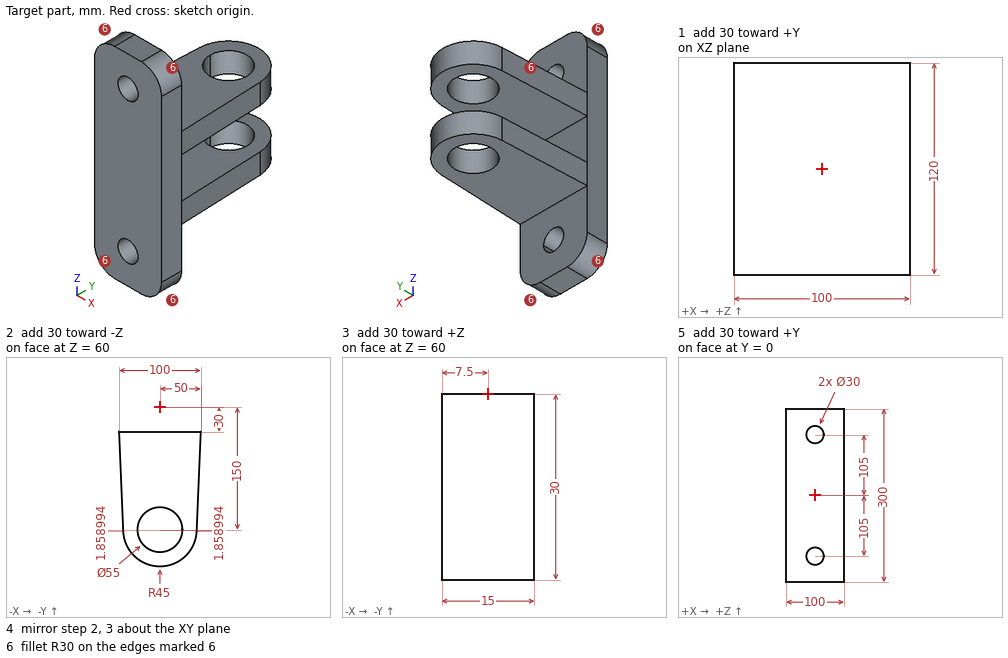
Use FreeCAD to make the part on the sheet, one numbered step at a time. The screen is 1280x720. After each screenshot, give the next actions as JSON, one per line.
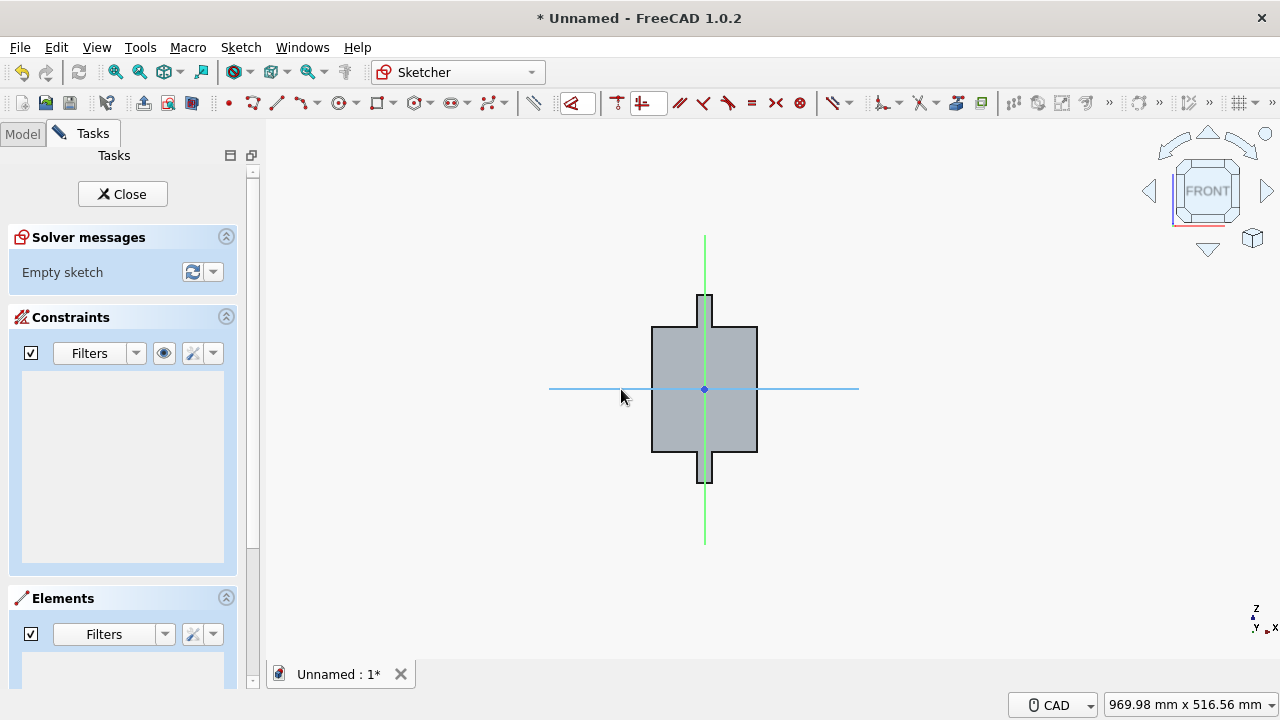
{"action": "left_click", "coordinate": [396, 104]}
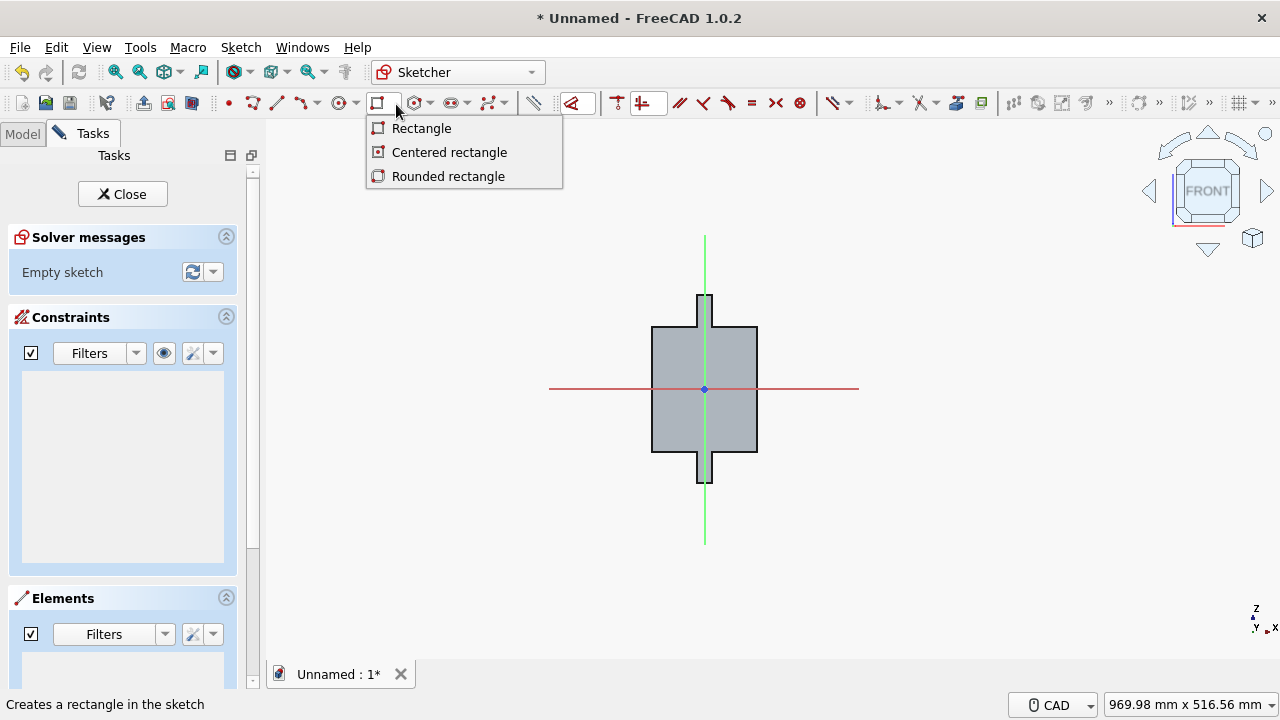
{"action": "left_click", "coordinate": [464, 152]}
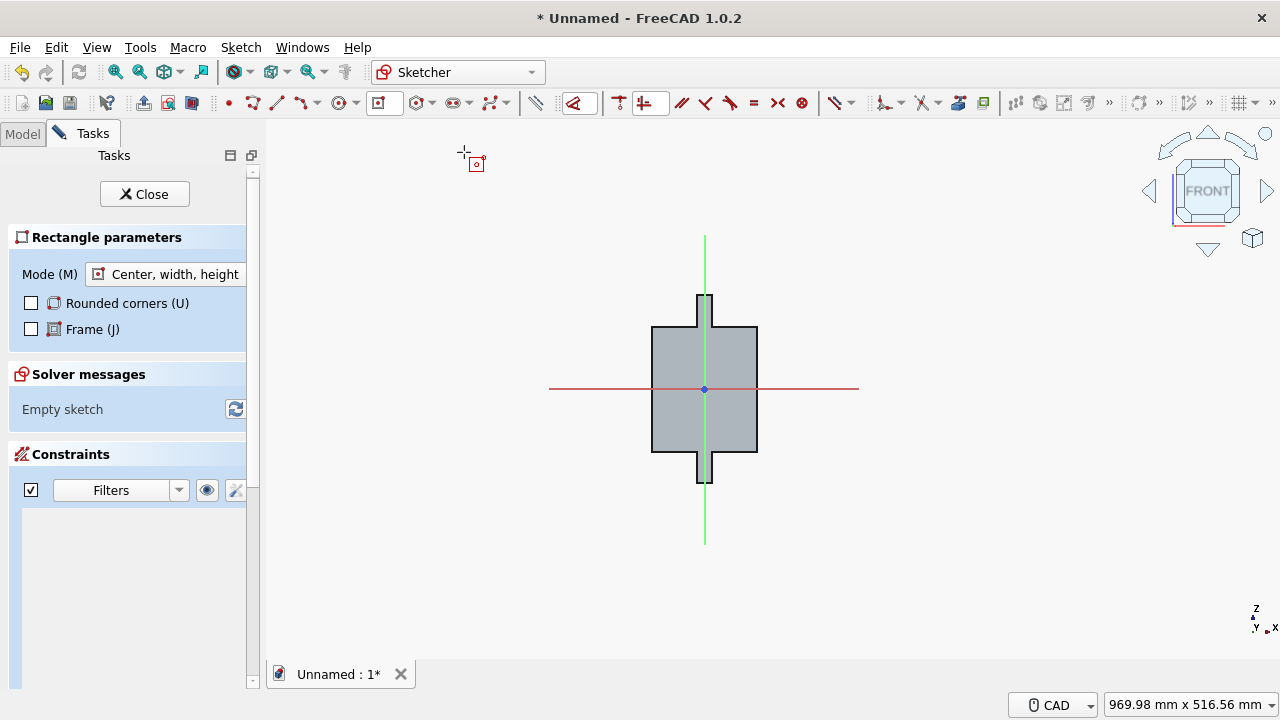
{"action": "left_click", "coordinate": [705, 389]}
{"action": "mouse_move", "coordinate": [757, 232]}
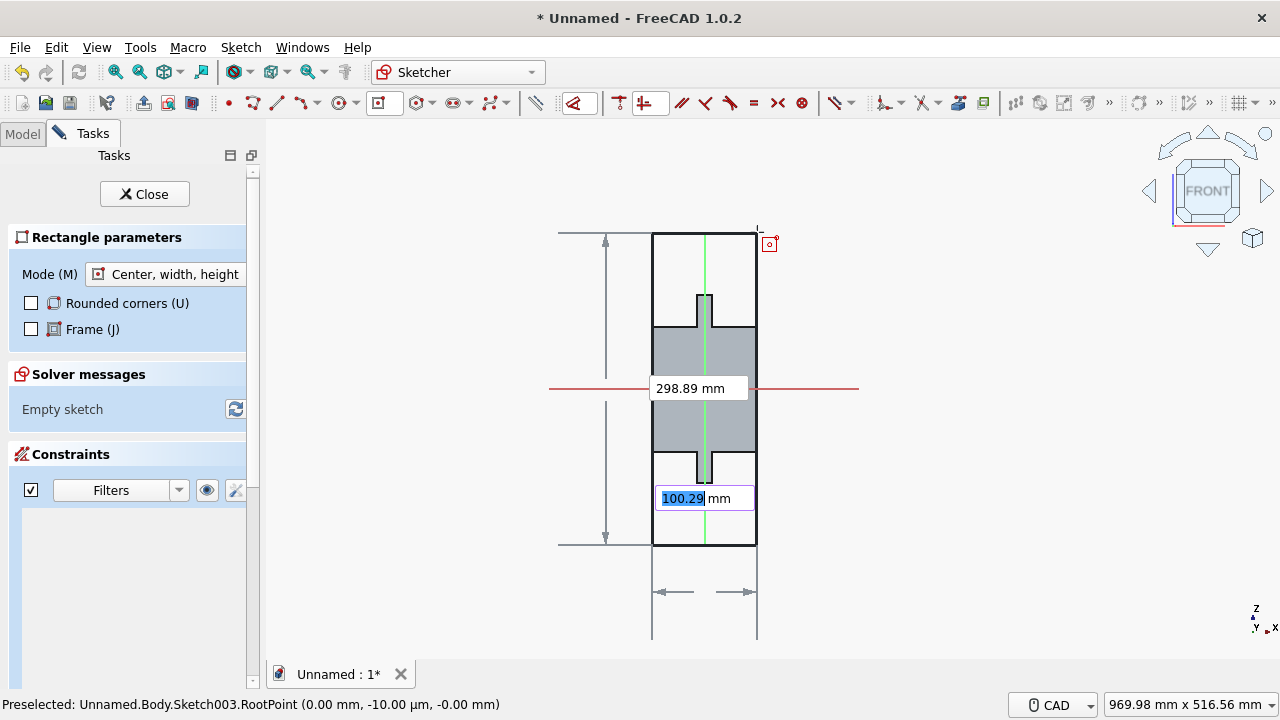
{"action": "type", "text": "100"}
{"action": "key", "text": "Tab"}
{"action": "type", "text": "300"}
{"action": "key", "text": "Return"}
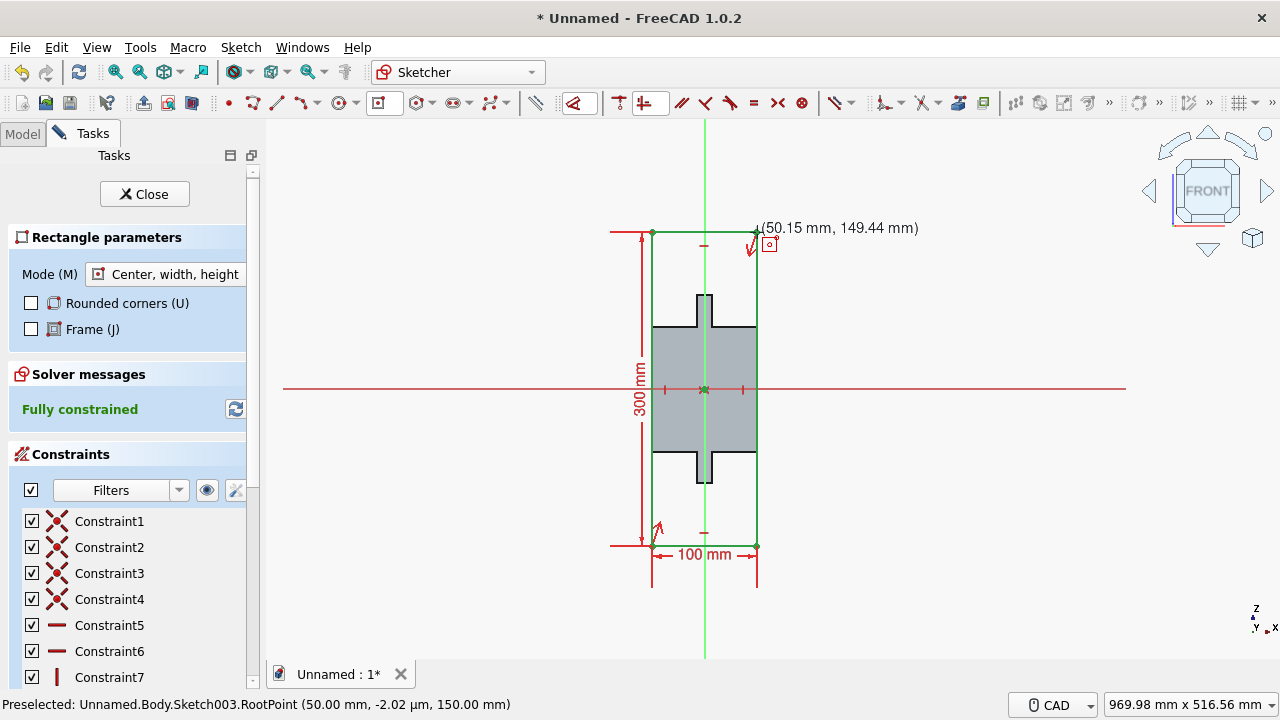
{"action": "key", "text": "g c"}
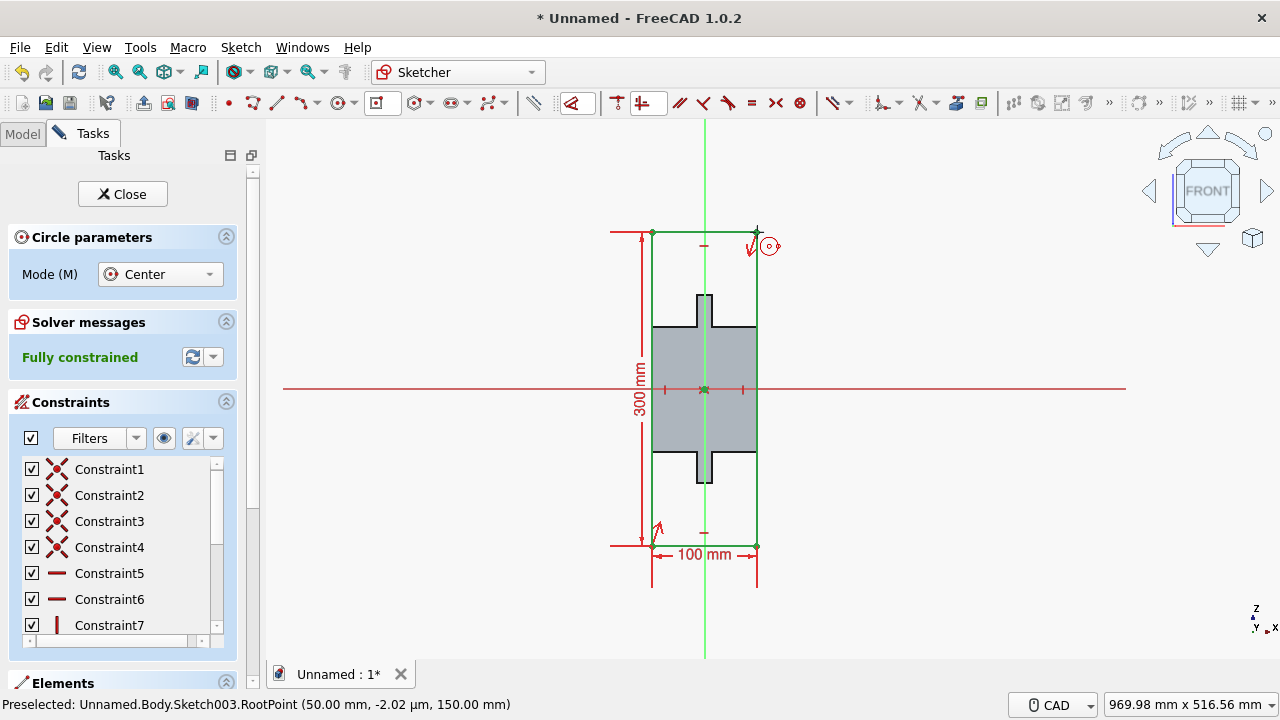
{"action": "scroll", "coordinate": [705, 499], "scroll_direction": "up", "scroll_amount": 2}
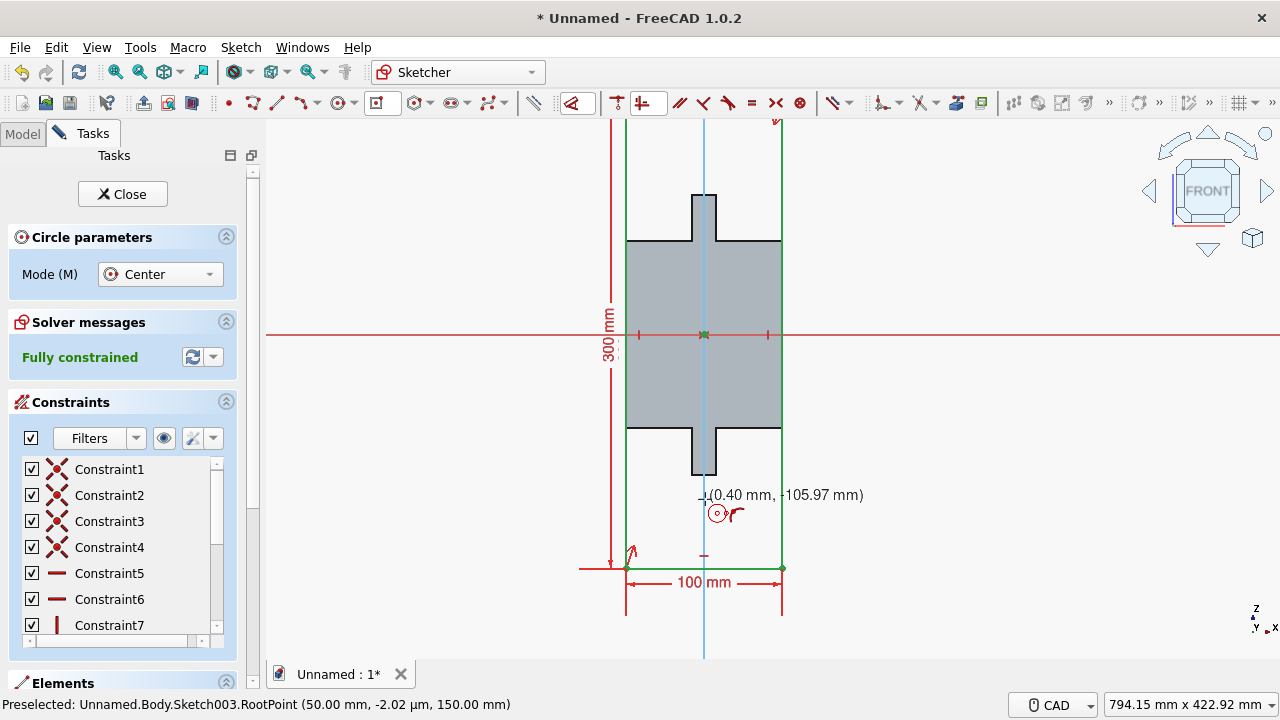
{"action": "left_click", "coordinate": [704, 499]}
{"action": "mouse_move", "coordinate": [721, 482]}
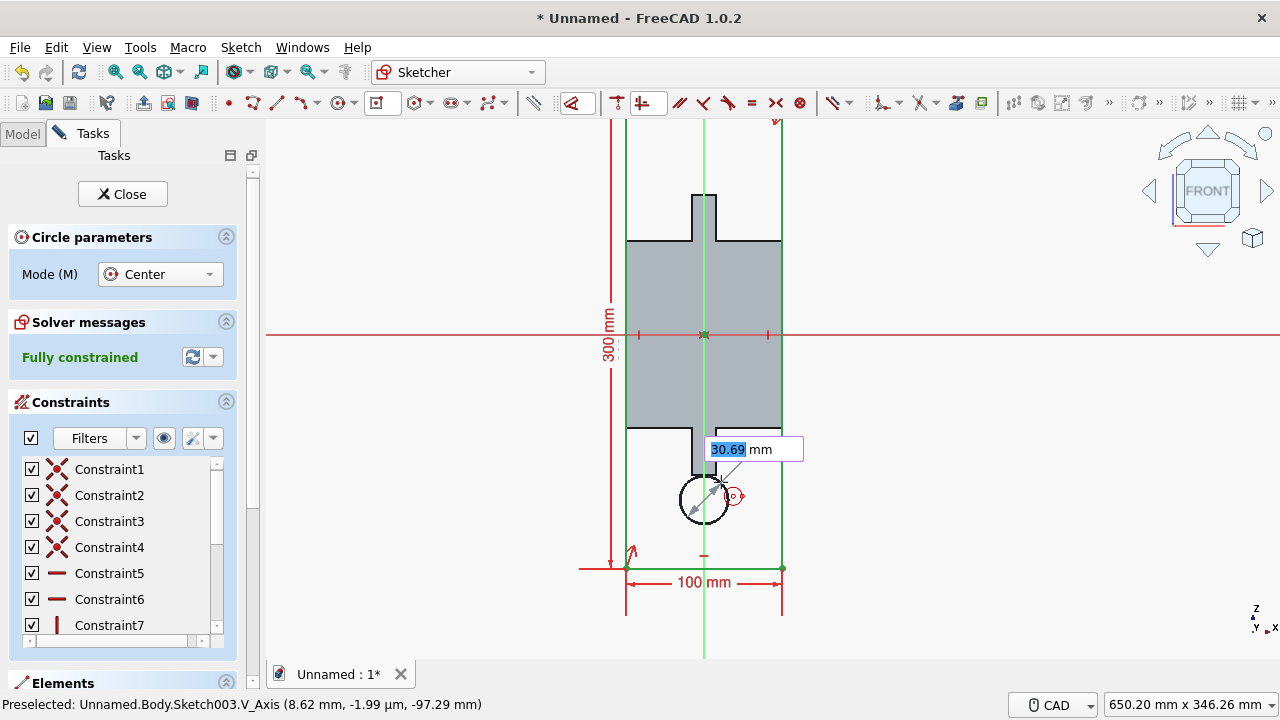
{"action": "type", "text": "30"}
{"action": "key", "text": "Return"}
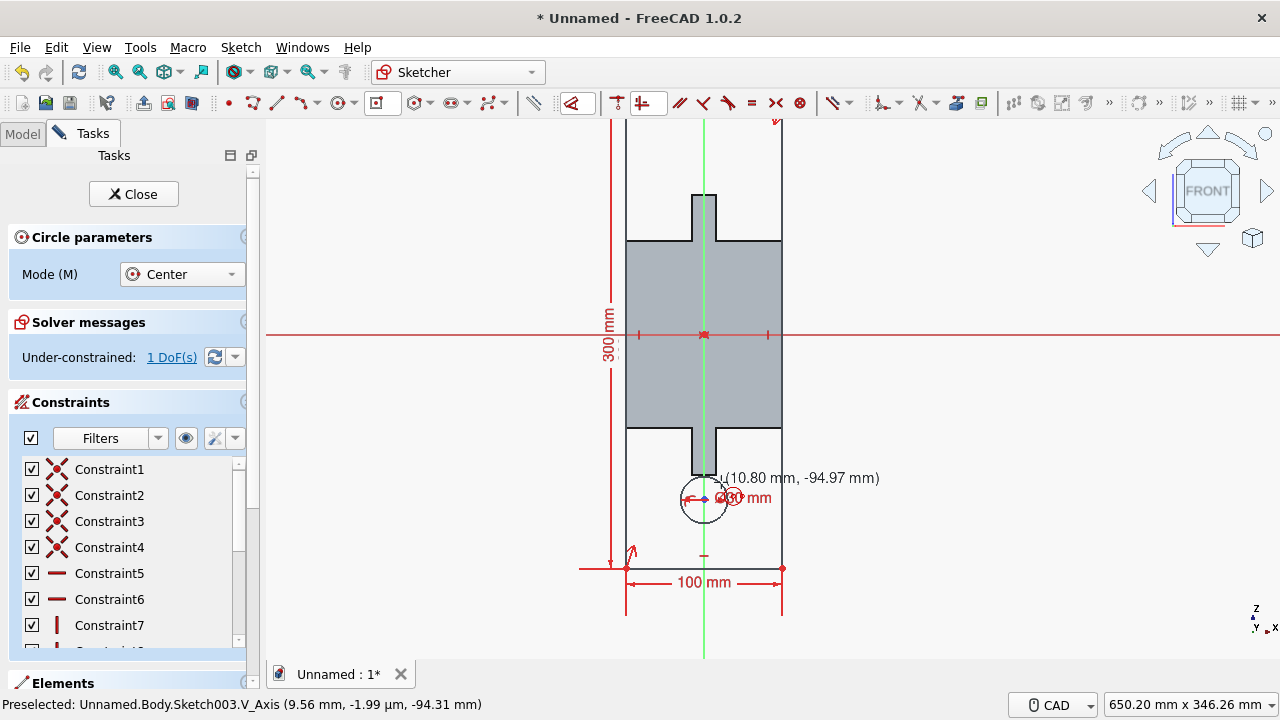
{"action": "left_click", "coordinate": [704, 171]}
{"action": "mouse_move", "coordinate": [721, 155]}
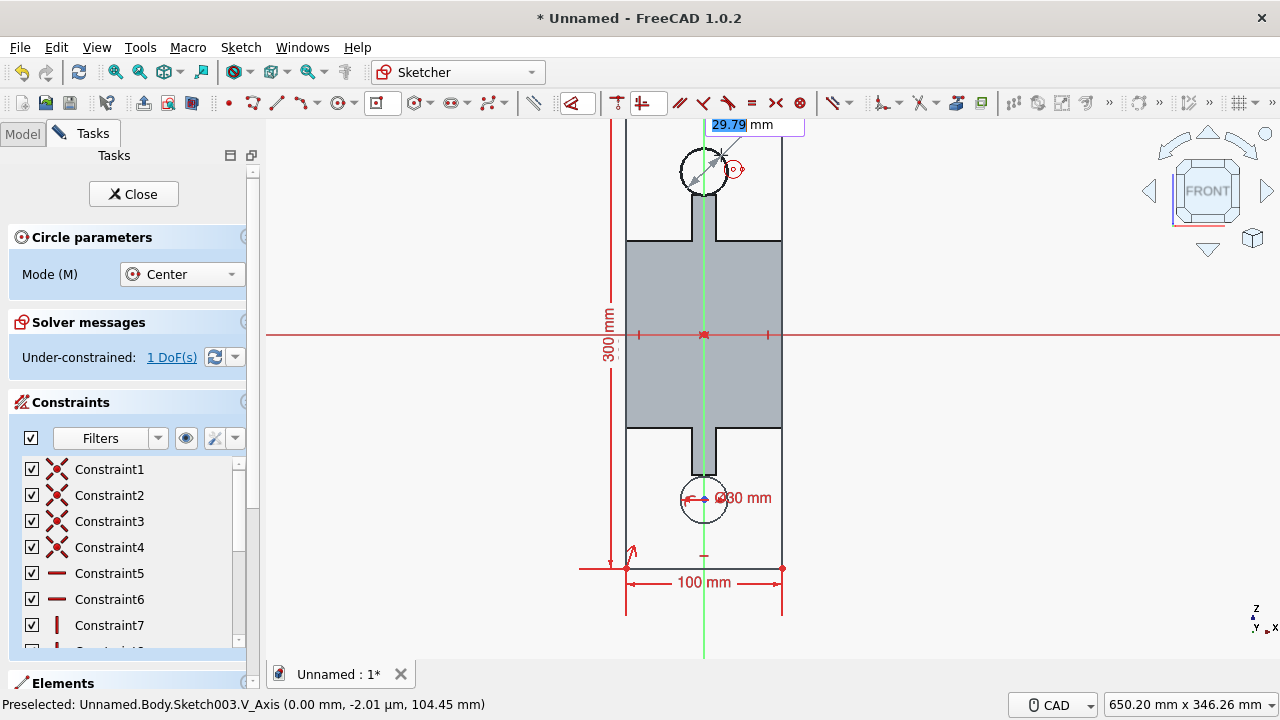
{"action": "type", "text": "30"}
{"action": "key", "text": "Return"}
{"action": "key", "text": "Escape"}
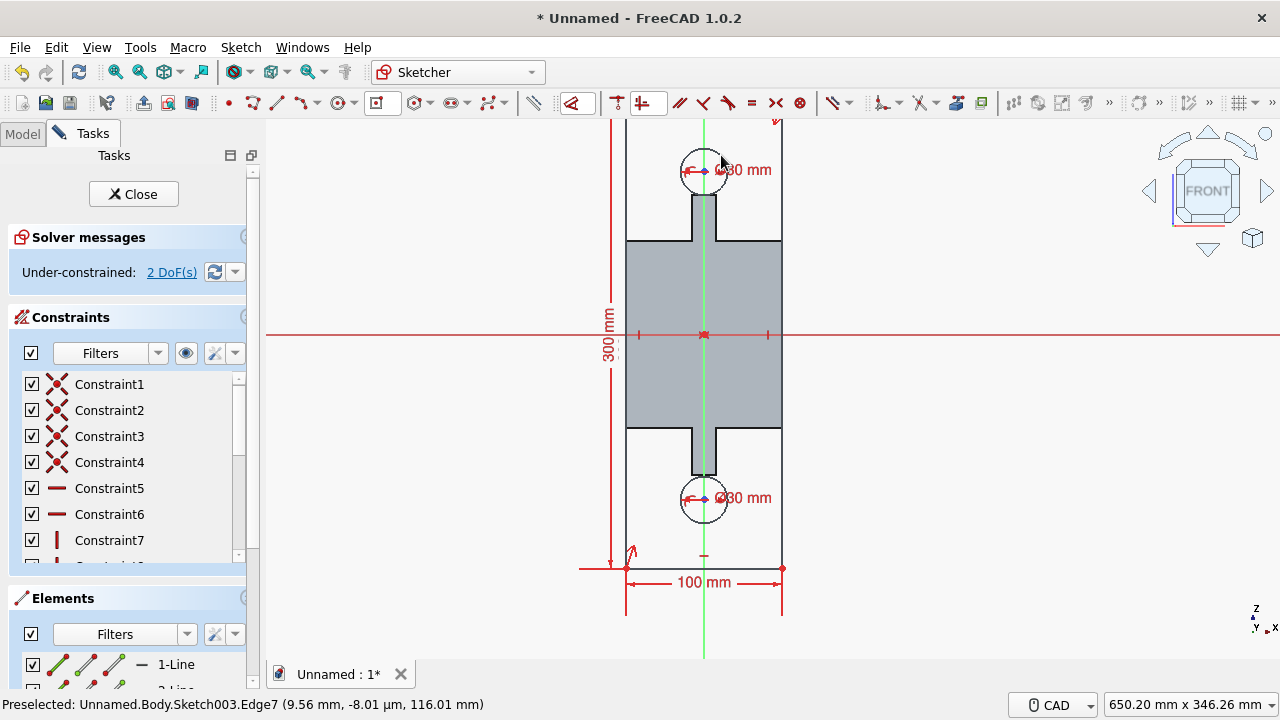
{"action": "left_click", "coordinate": [704, 500]}